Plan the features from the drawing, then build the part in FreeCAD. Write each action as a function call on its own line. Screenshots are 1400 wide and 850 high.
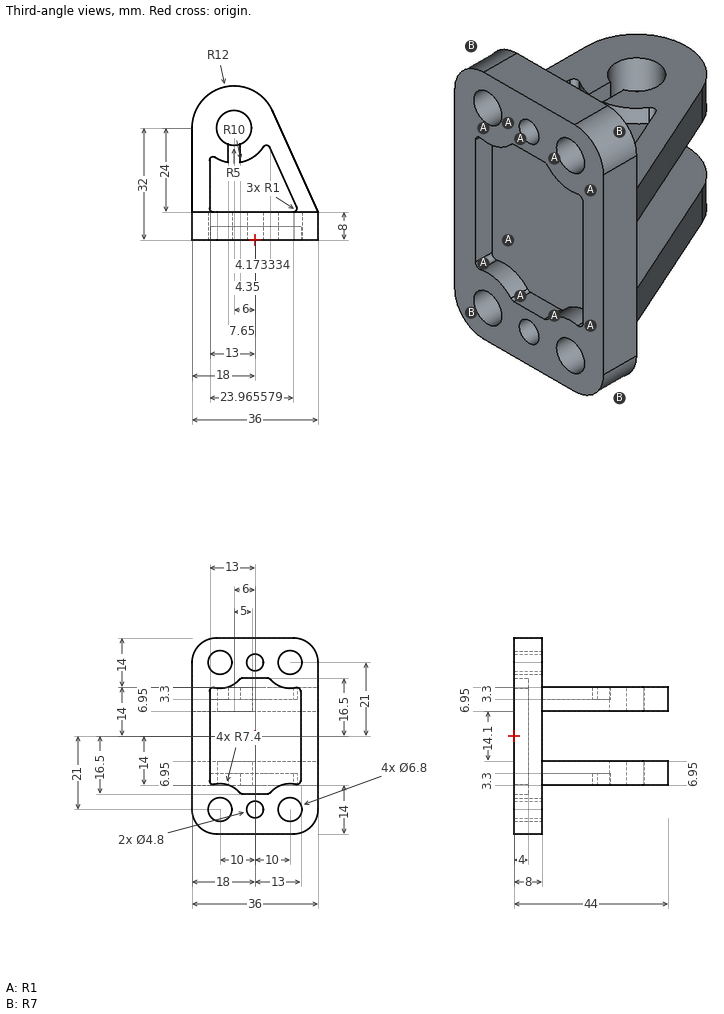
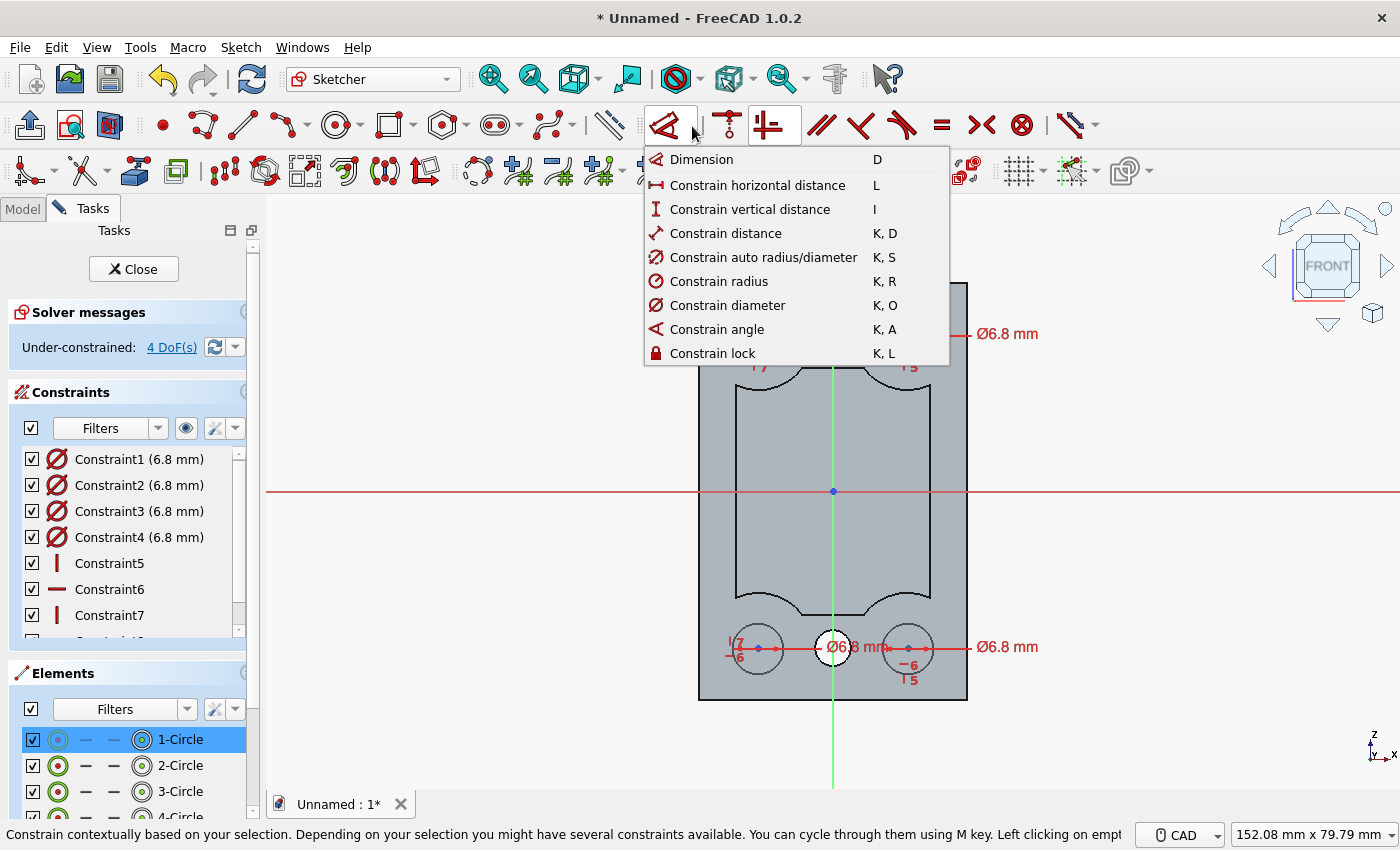
click(797, 185)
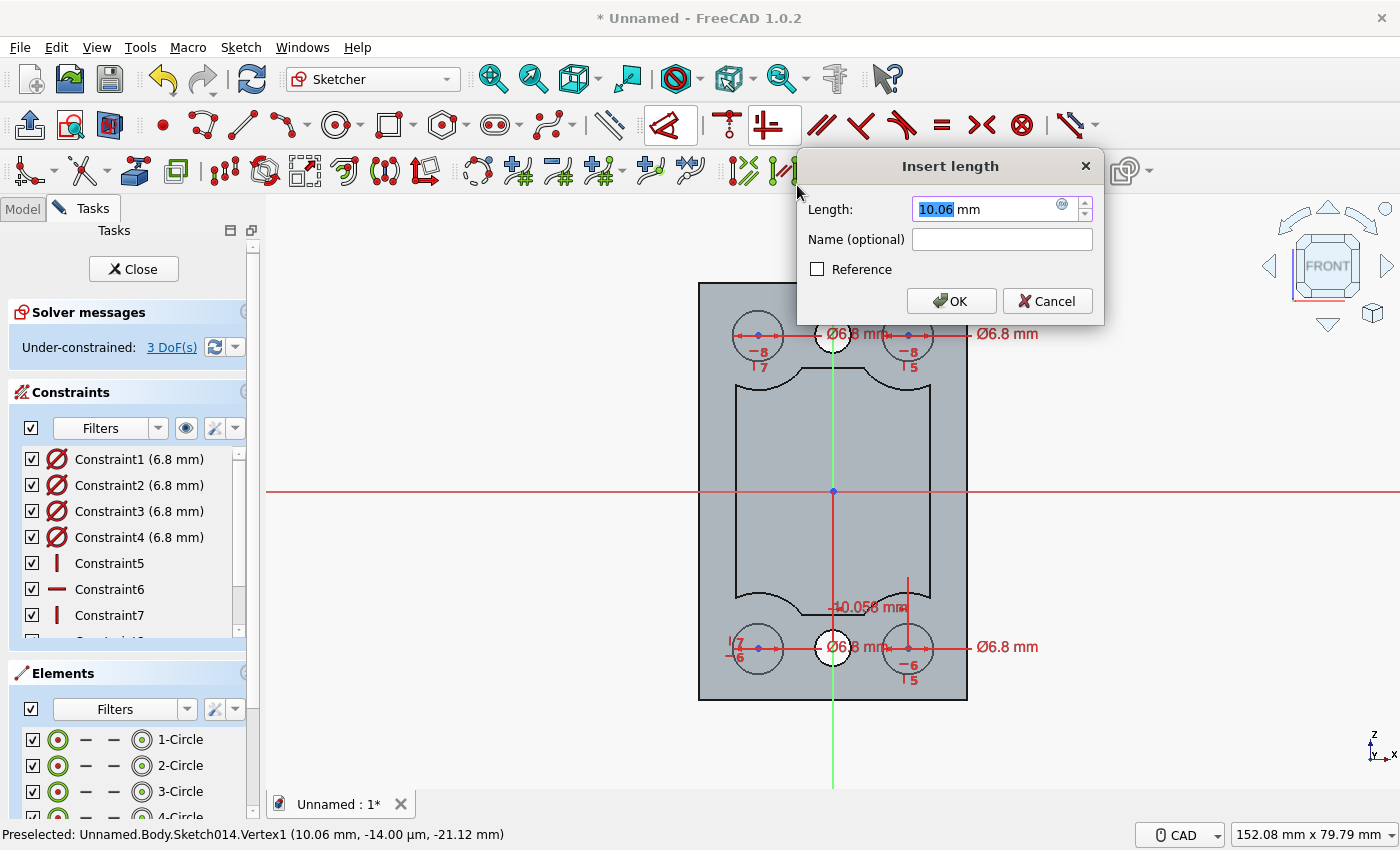
text(10)
key(Return)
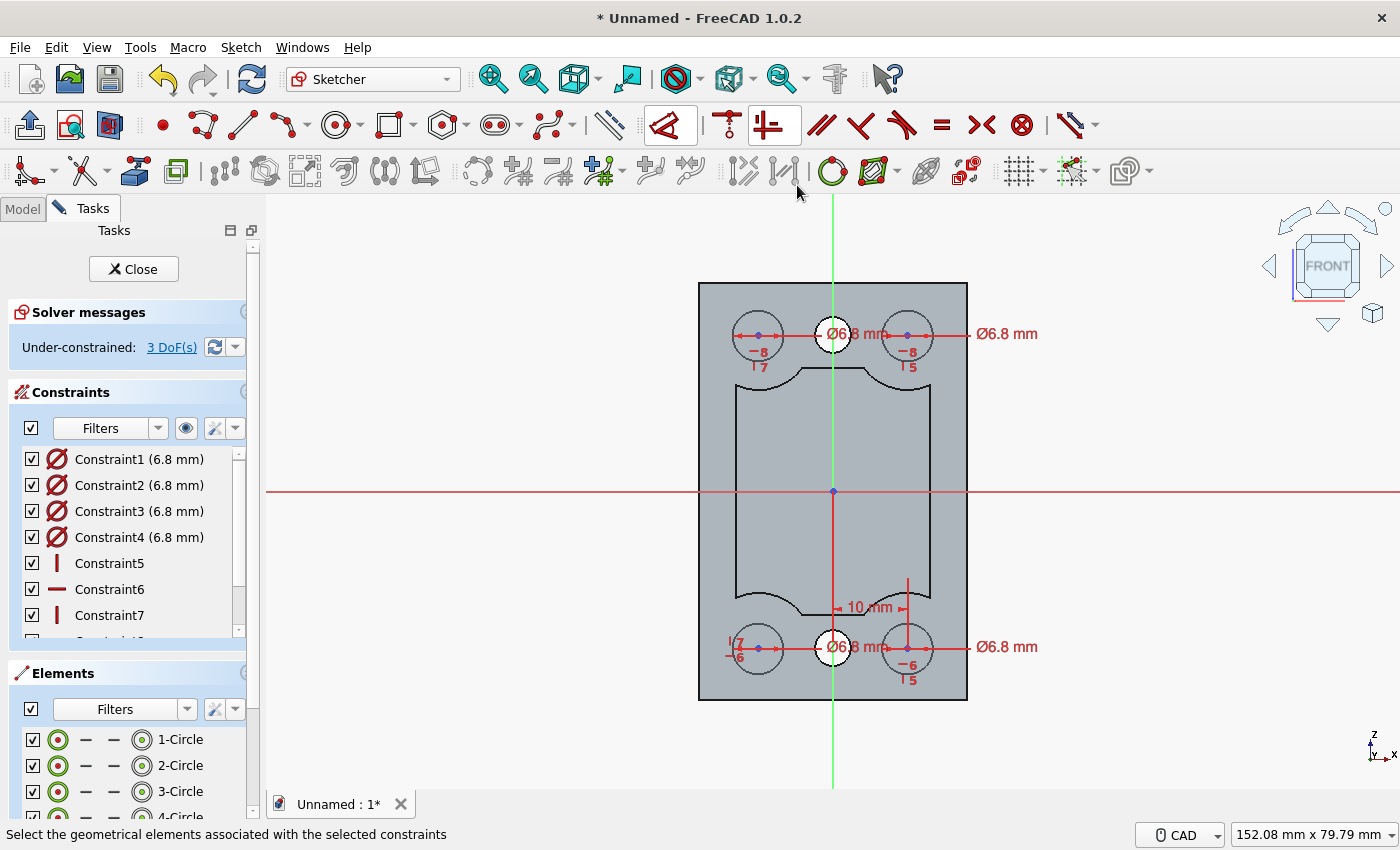
click(908, 649)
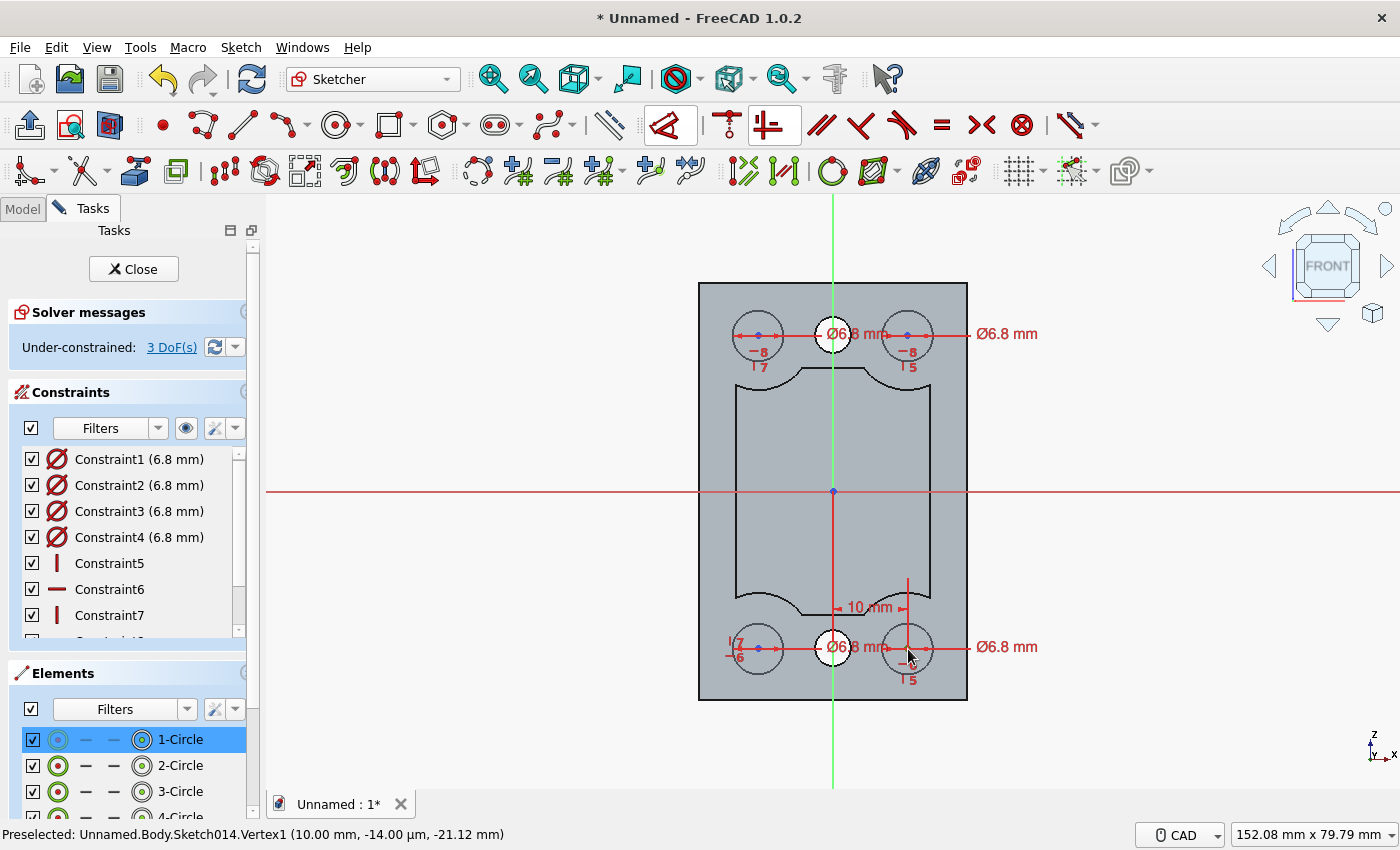
key(i)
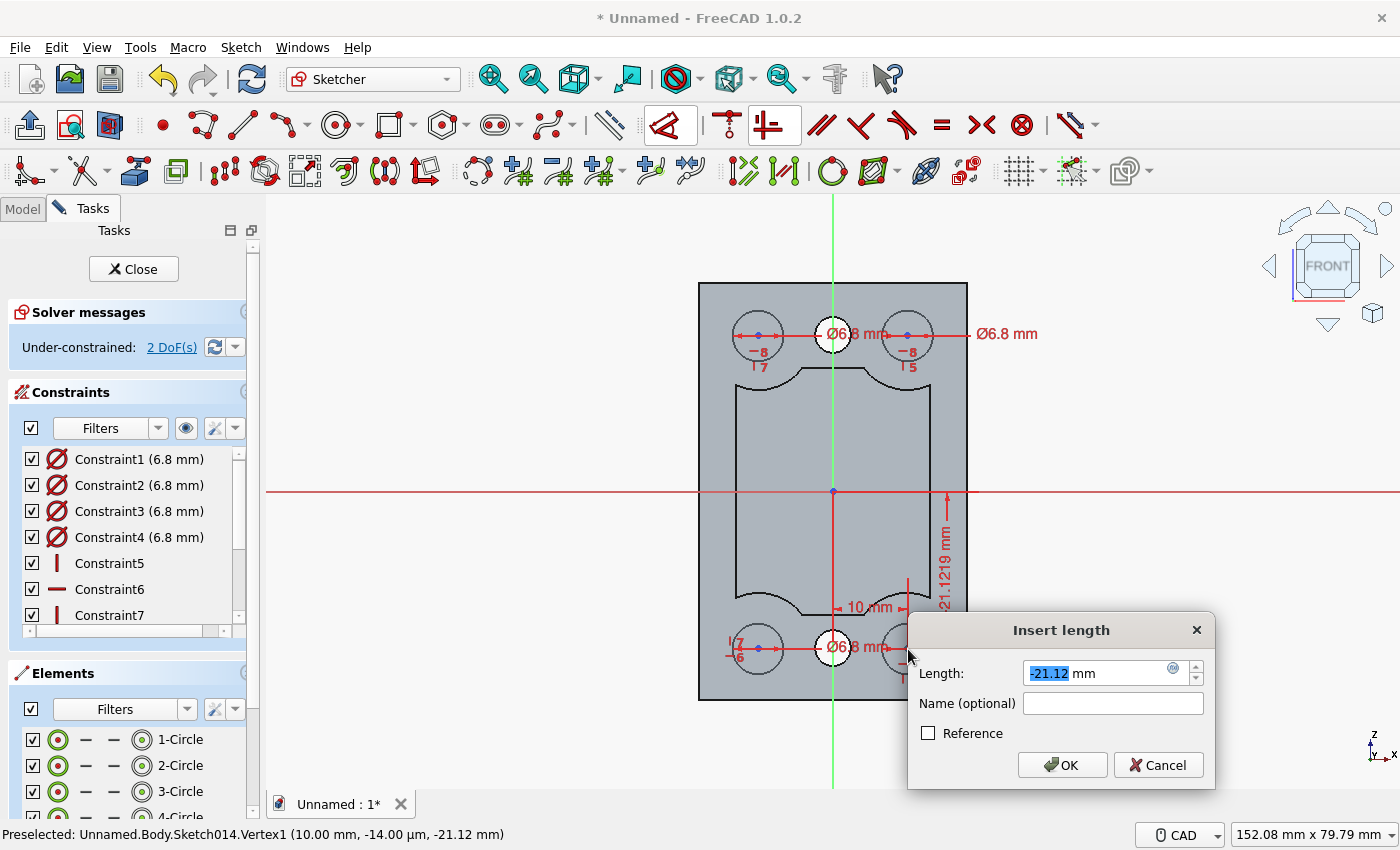
text(-21)
key(Return)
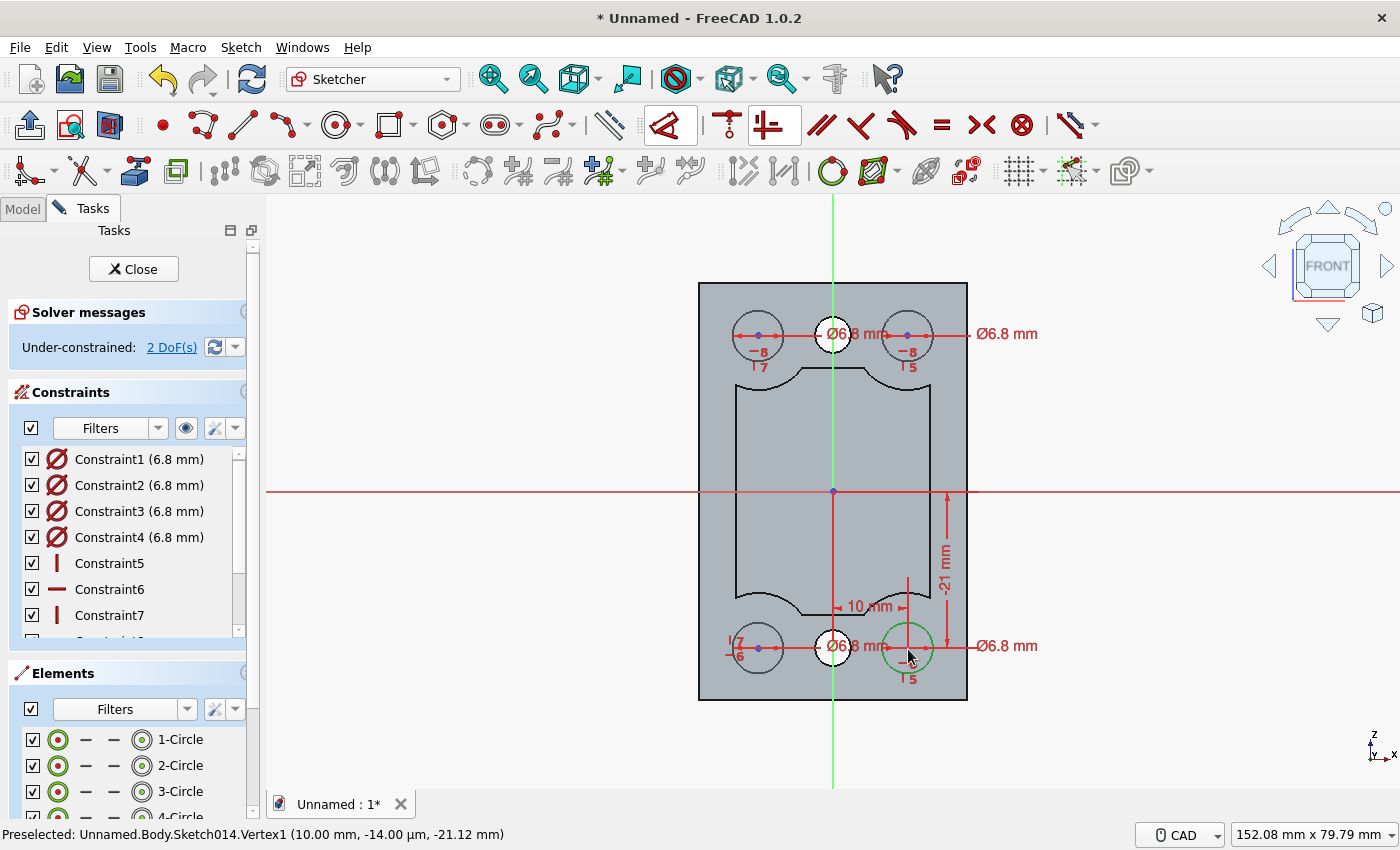
click(908, 336)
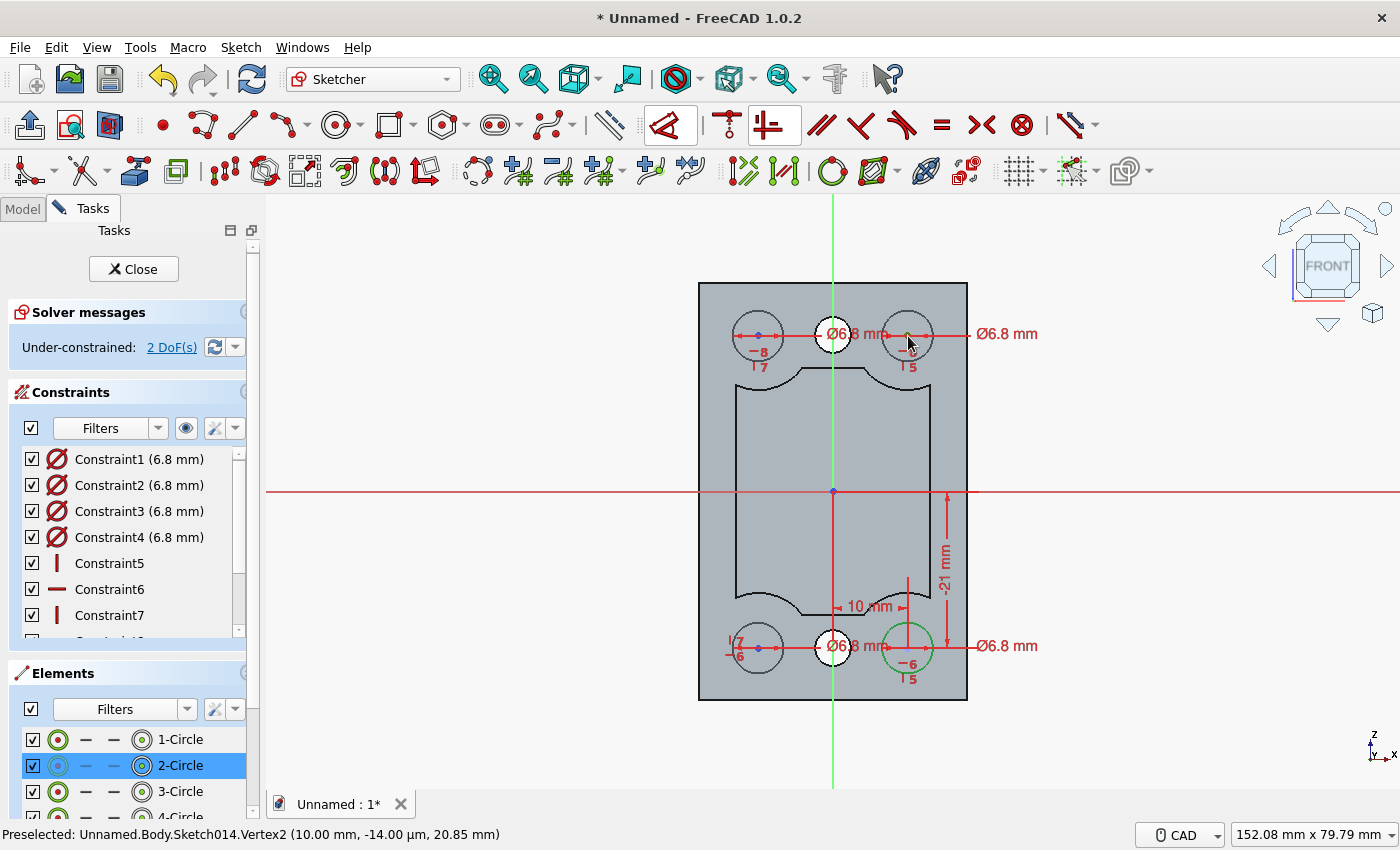
key(i)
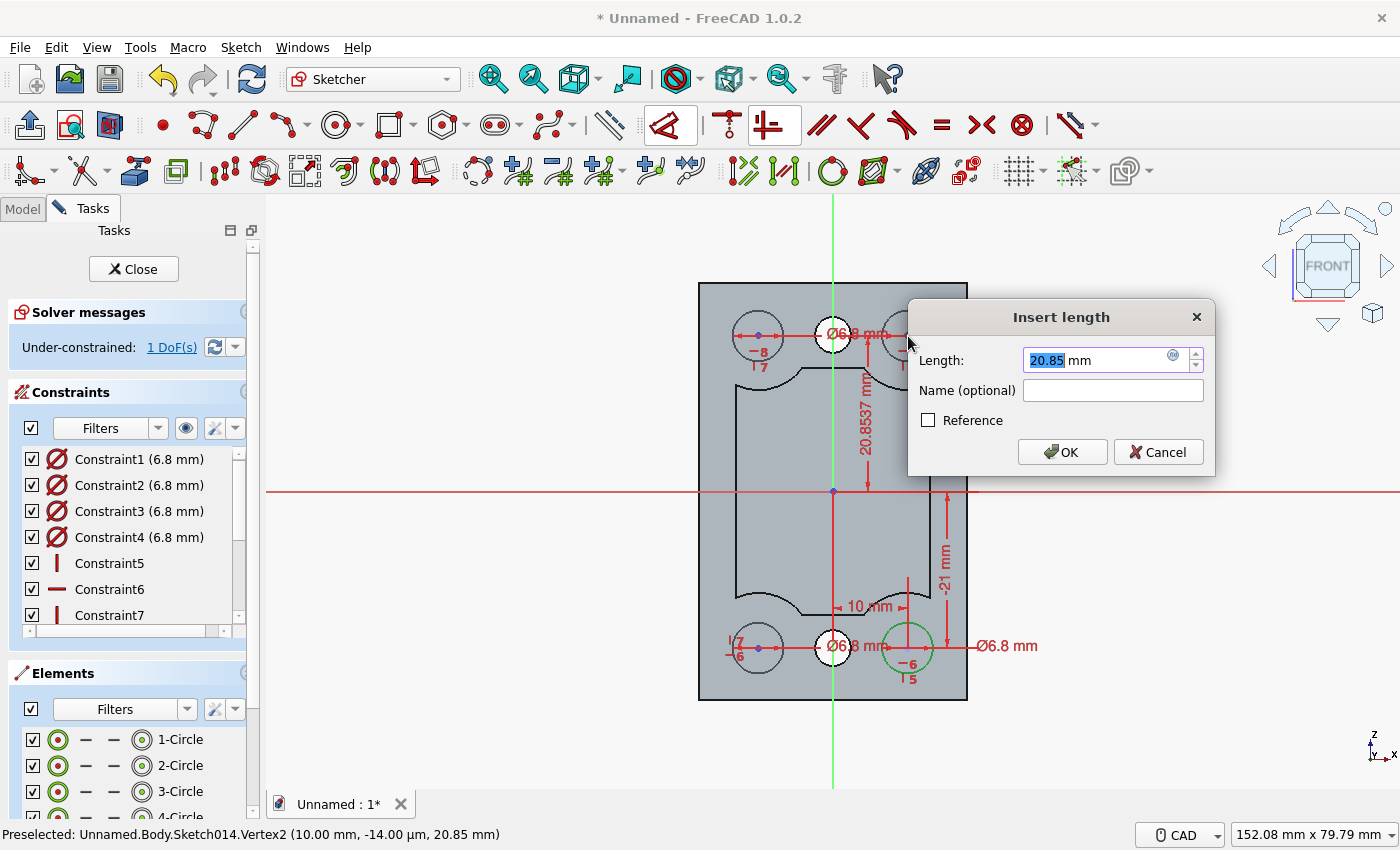
text(21)
key(Return)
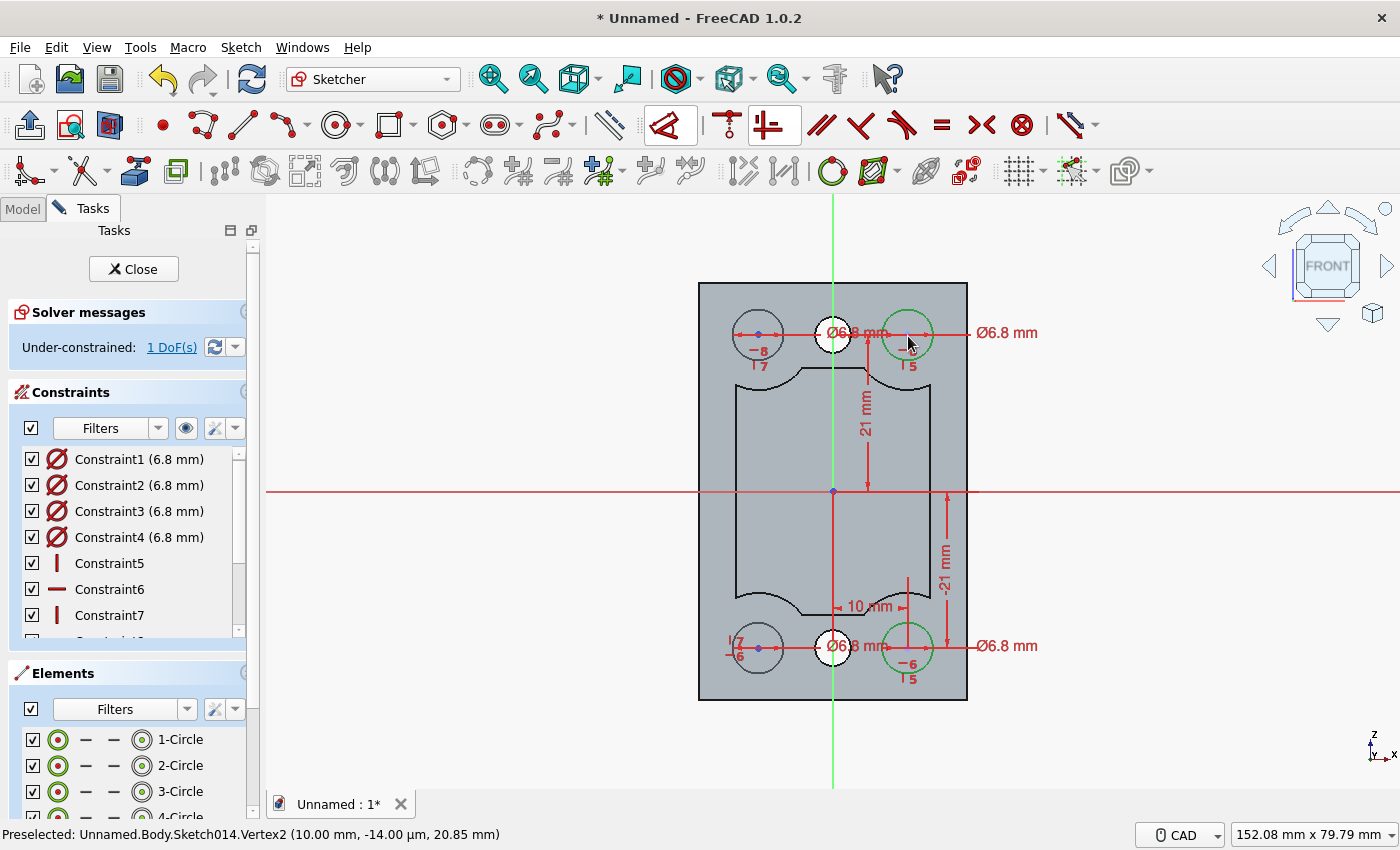
click(758, 648)